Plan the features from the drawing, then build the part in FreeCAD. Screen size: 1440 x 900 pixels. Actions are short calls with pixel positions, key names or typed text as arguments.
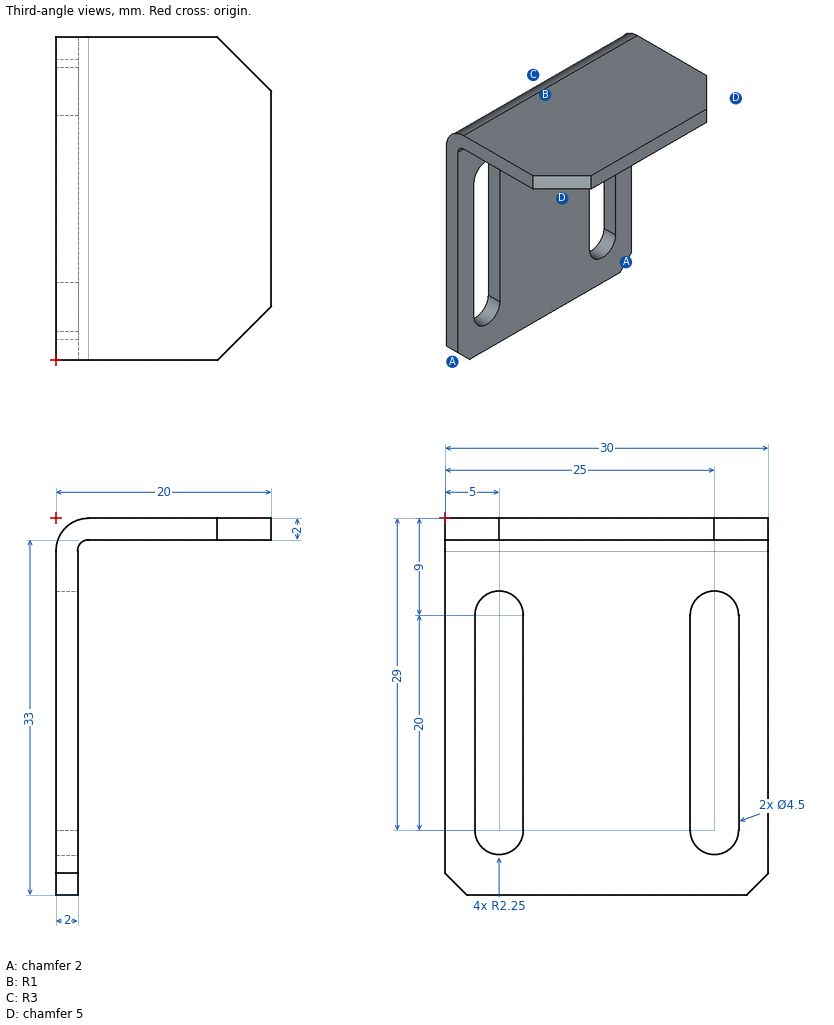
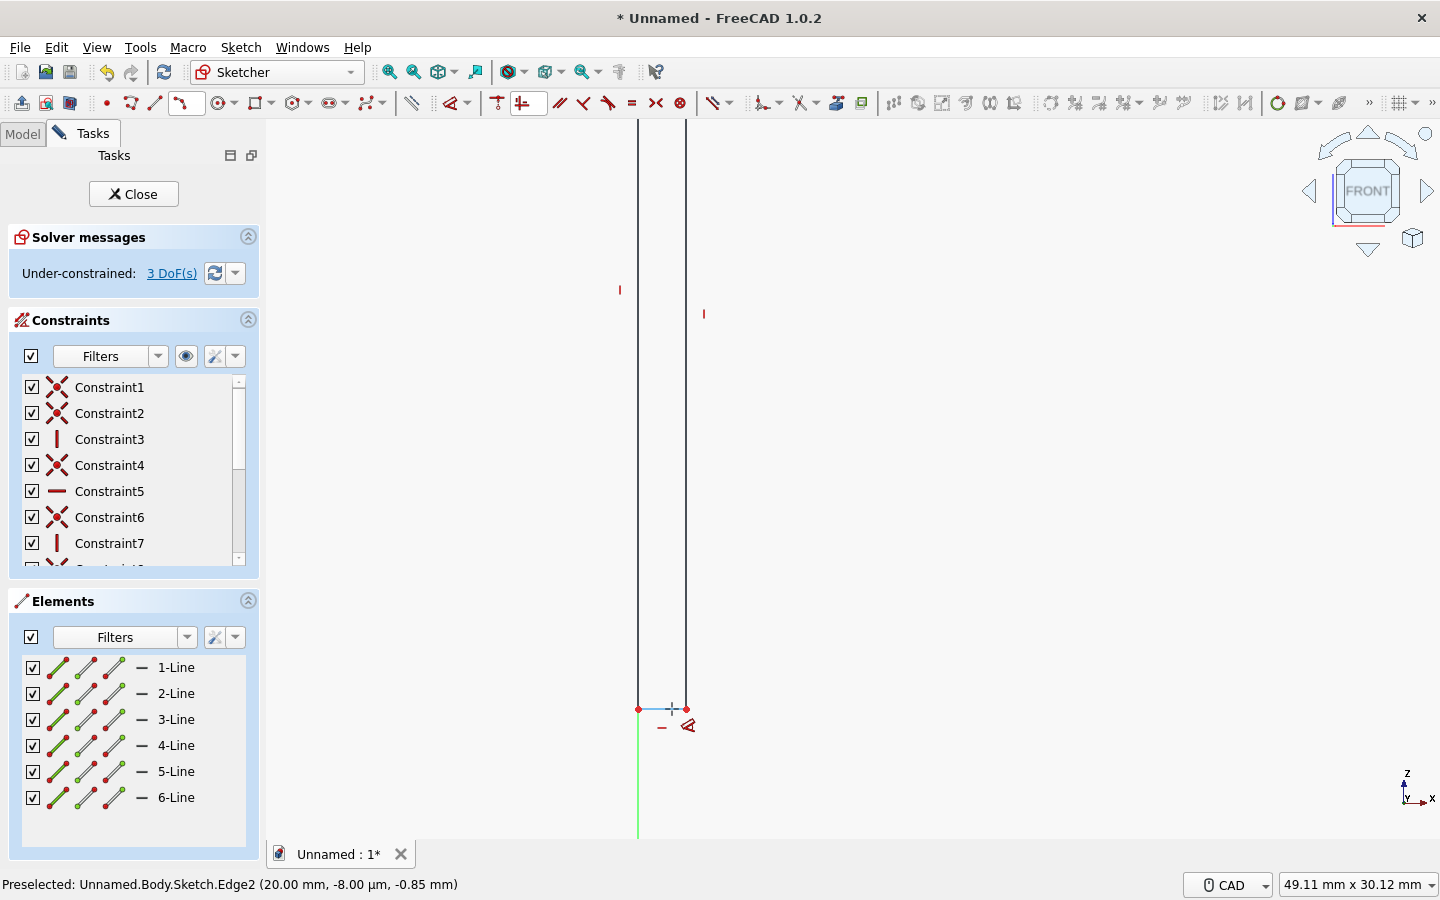
click(672, 709)
click(662, 743)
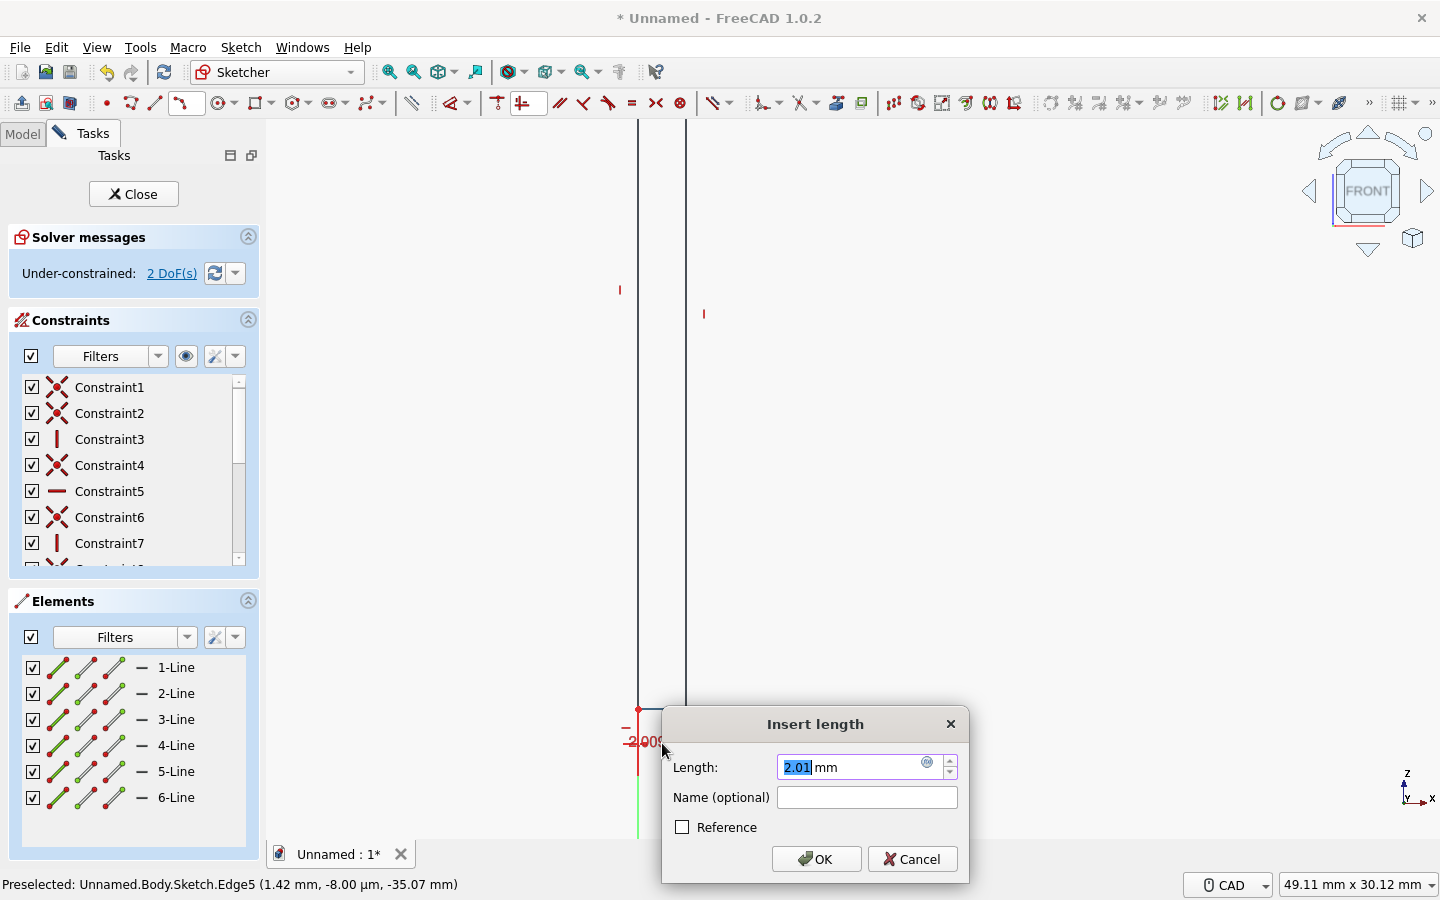
text(2)
key(Return)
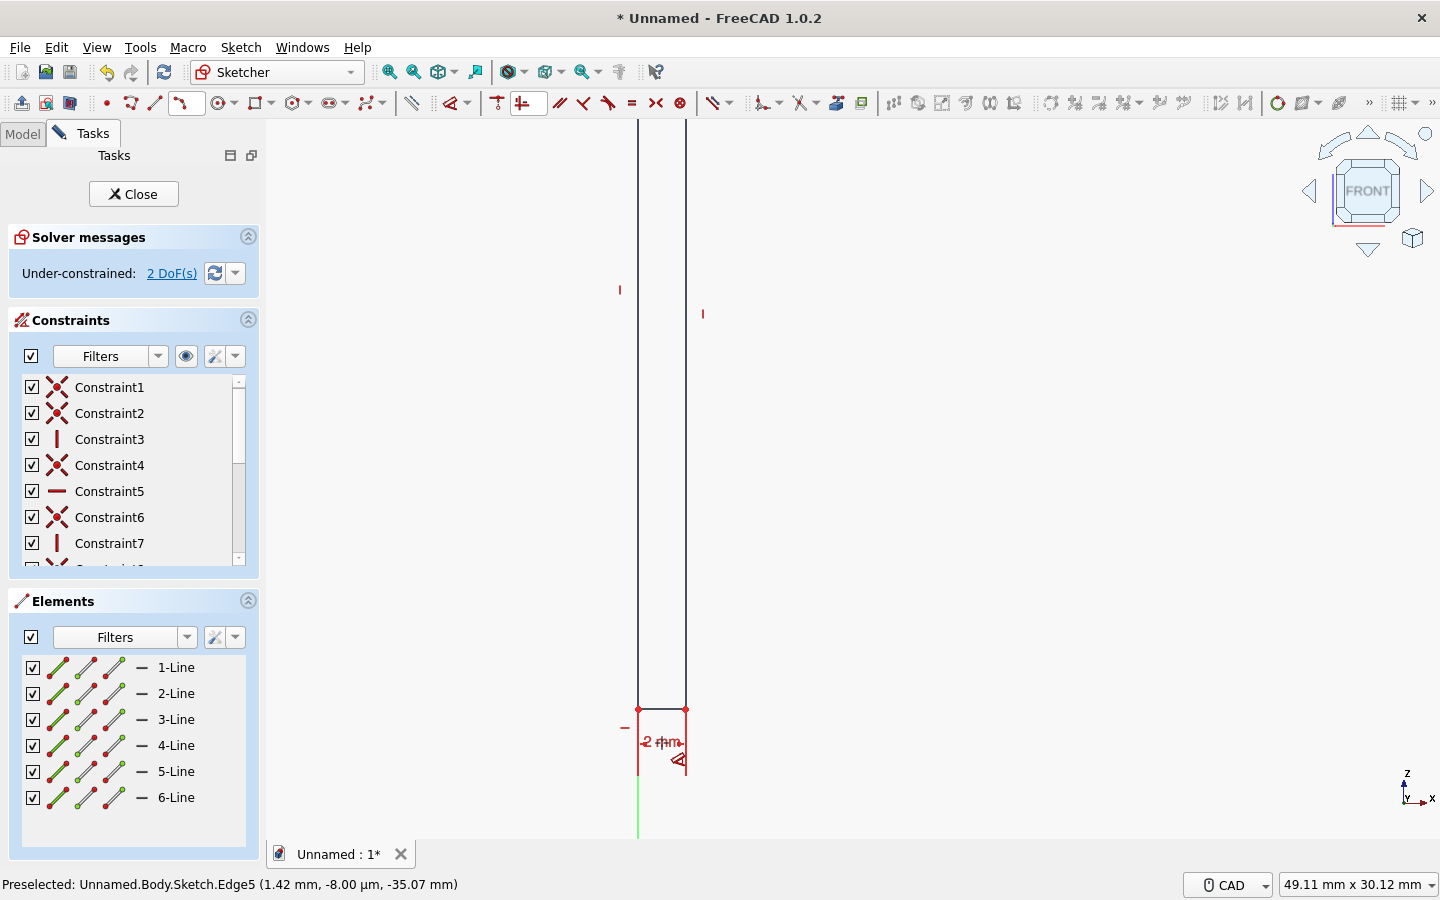
scroll(672, 710, down, 3)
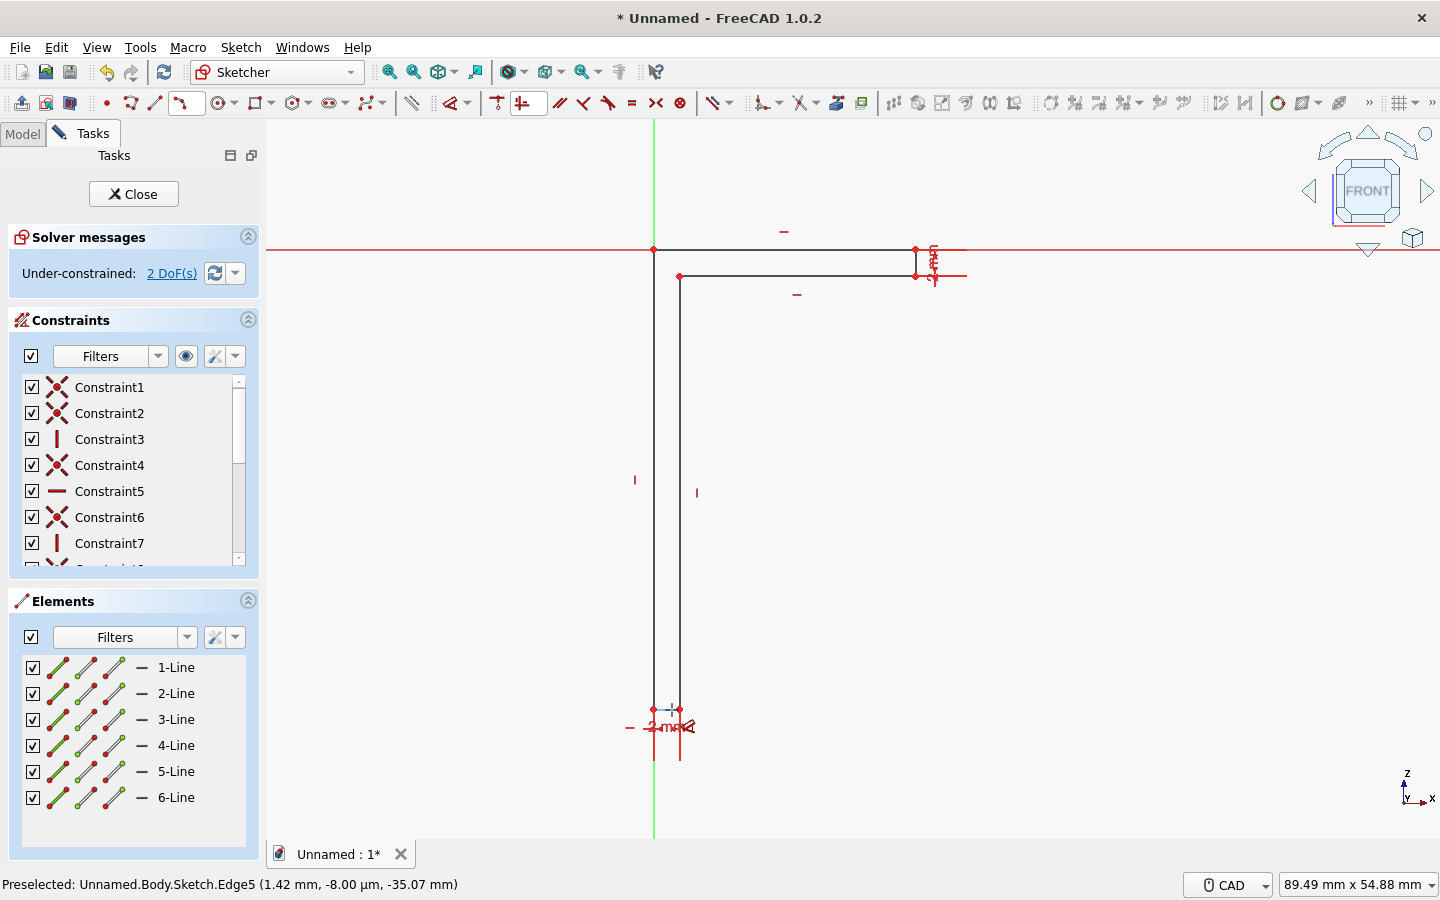
click(732, 250)
click(785, 216)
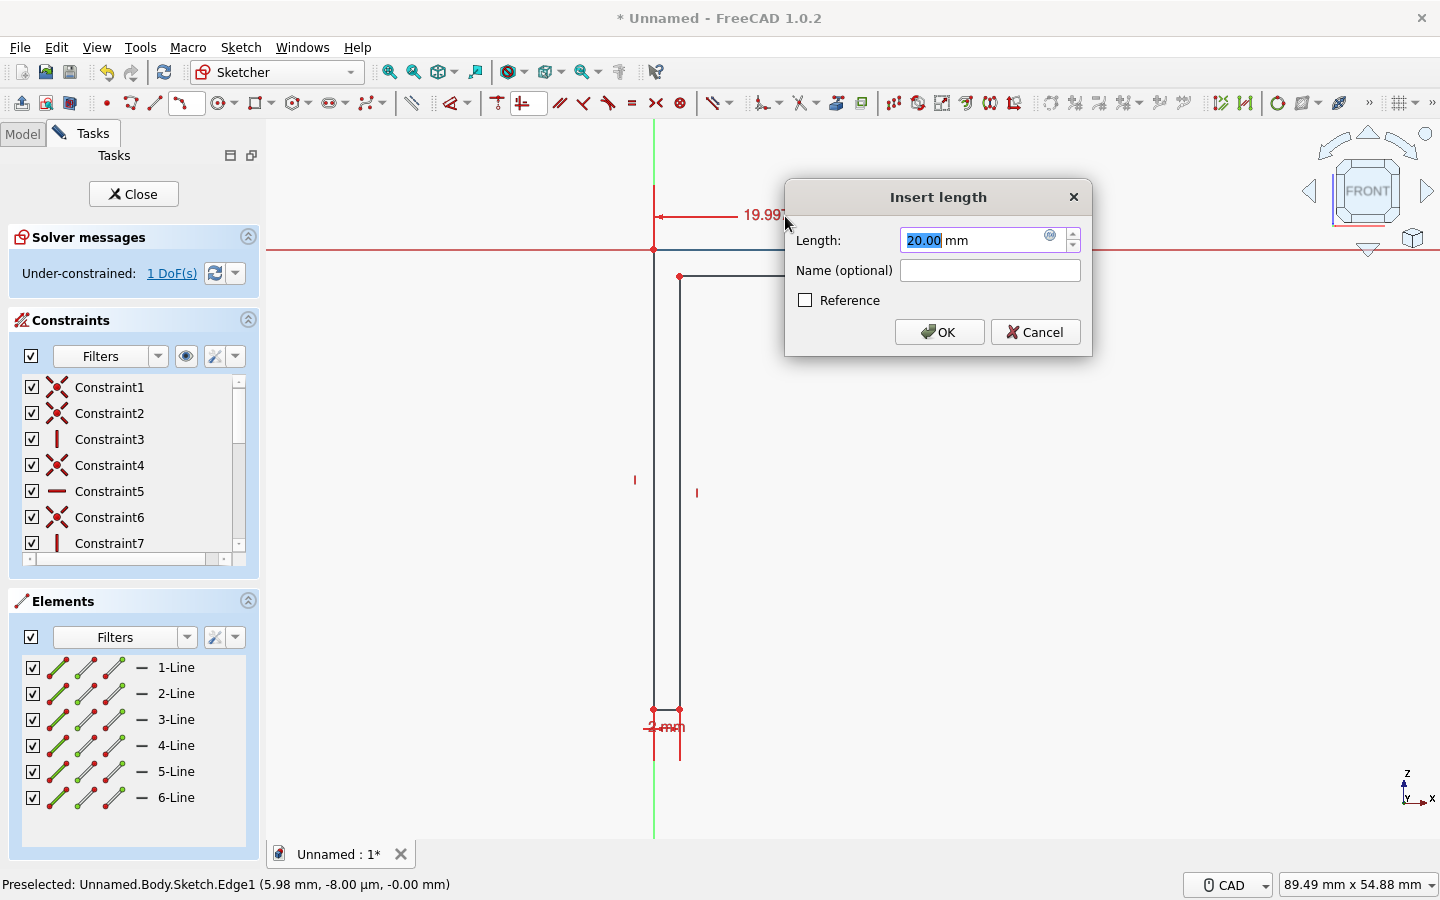
text(20)
key(Return)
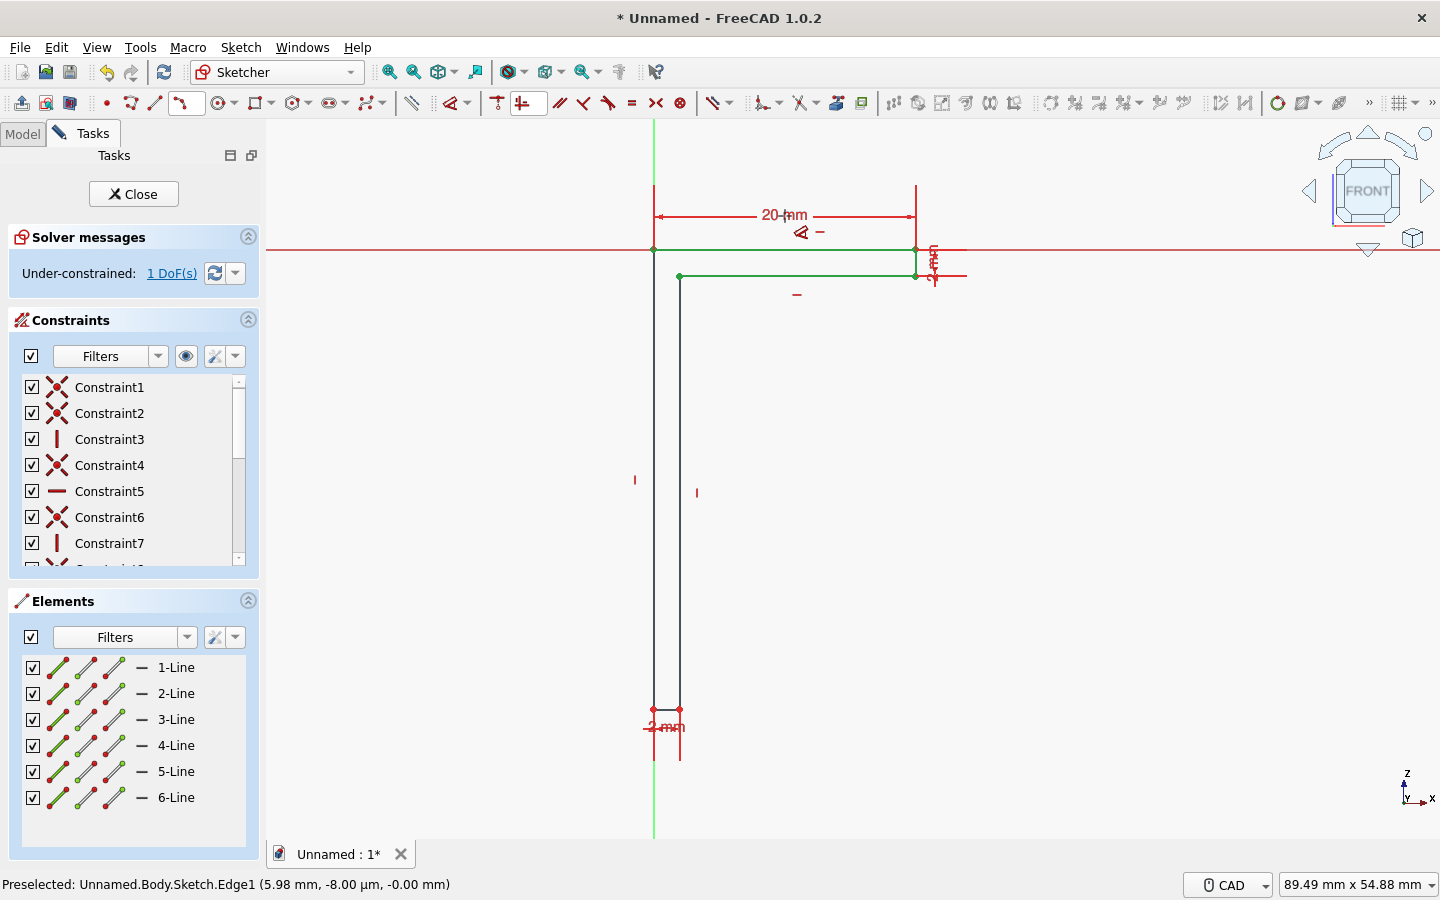
click(680, 406)
click(714, 493)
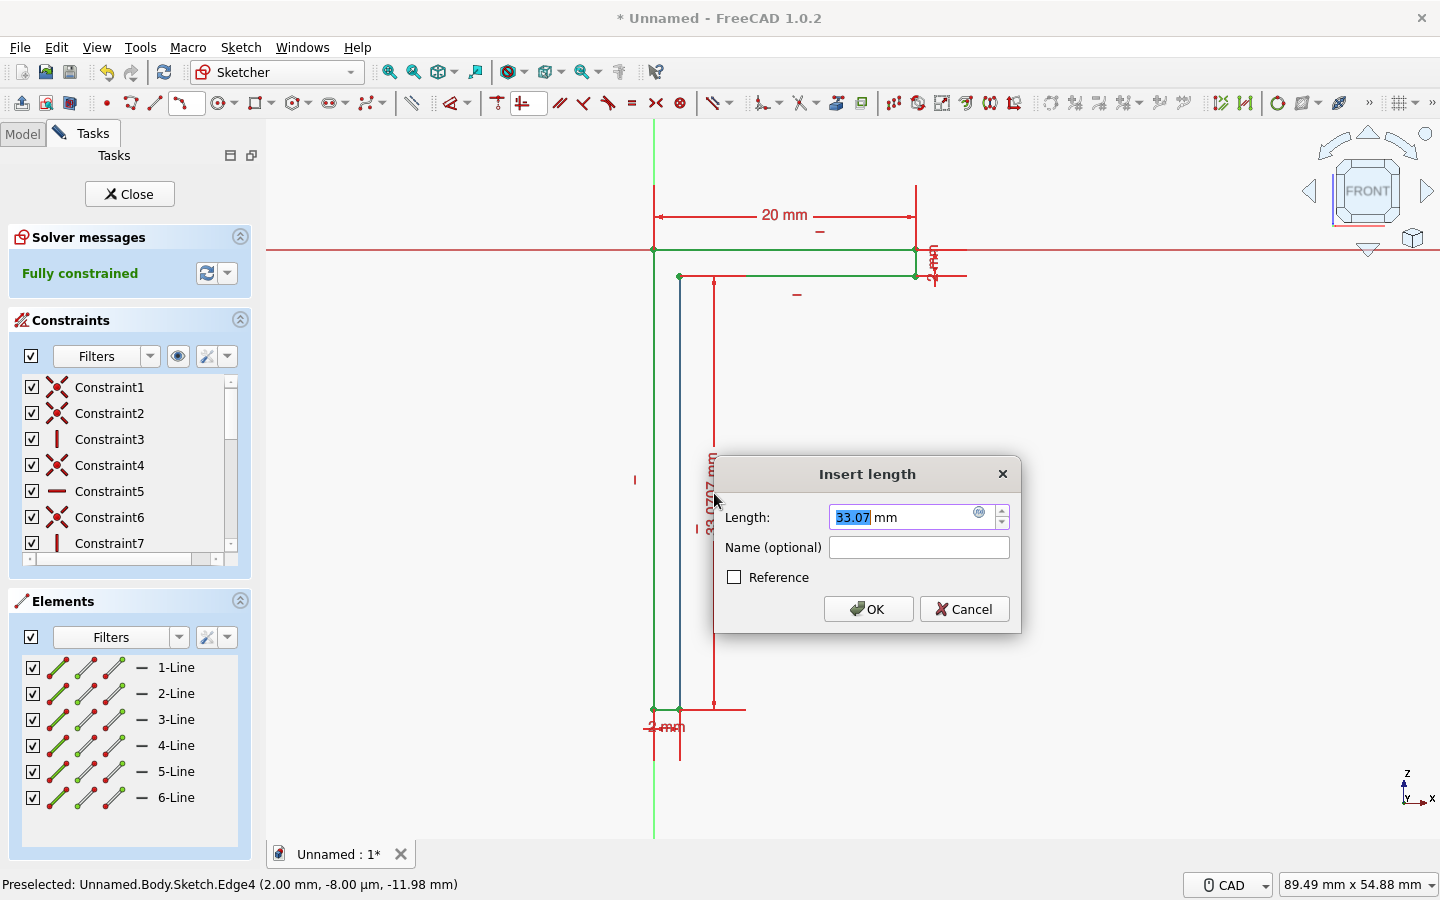
text(33)
key(Return)
key(Escape)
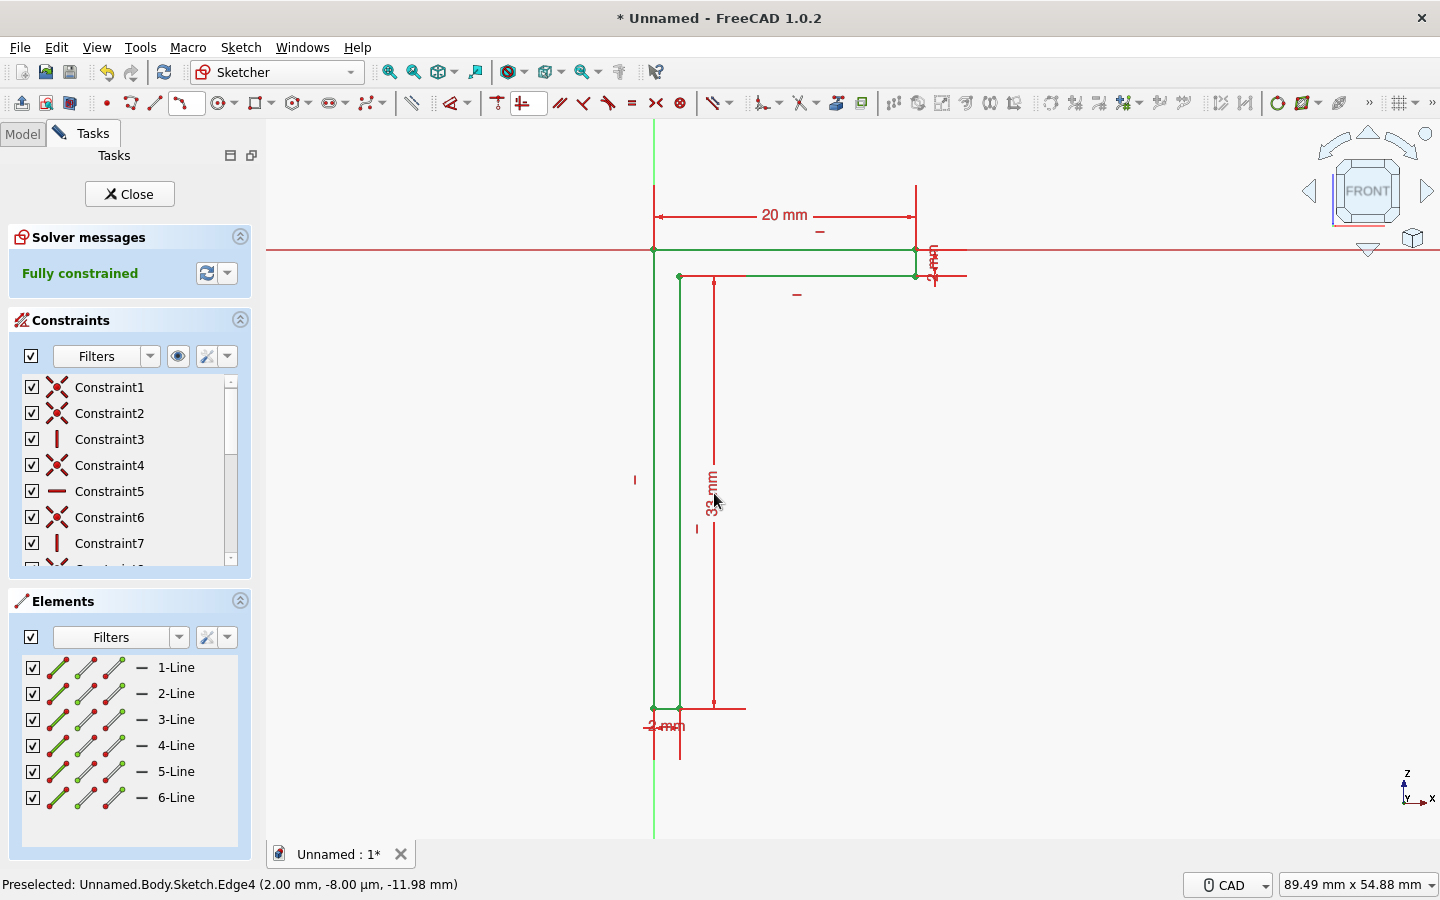
click(130, 194)